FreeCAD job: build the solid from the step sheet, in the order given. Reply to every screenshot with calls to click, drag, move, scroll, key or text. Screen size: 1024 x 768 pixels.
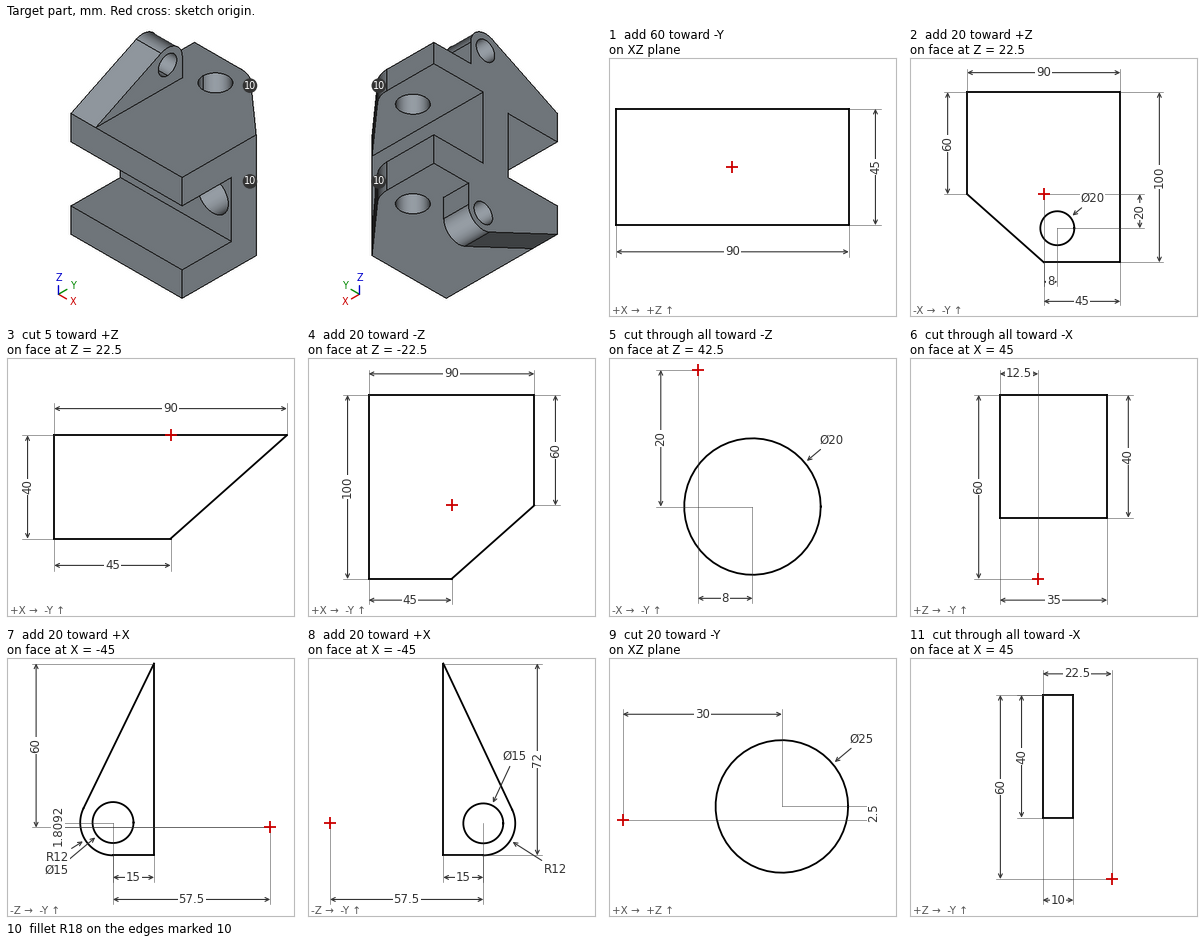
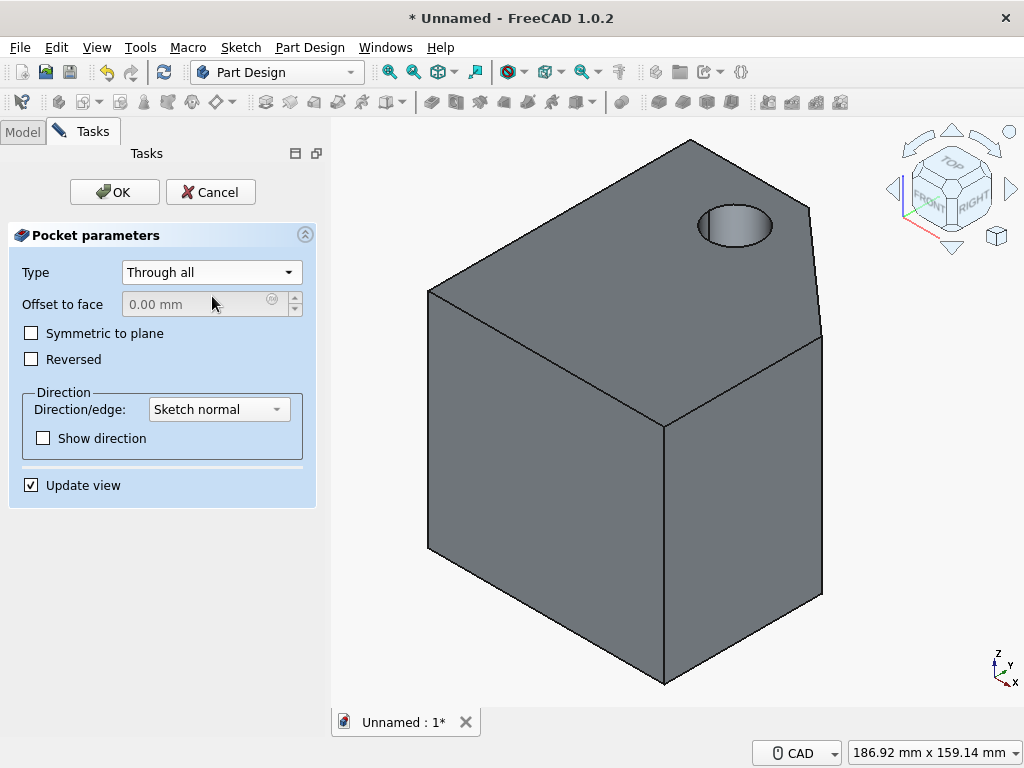
click(115, 192)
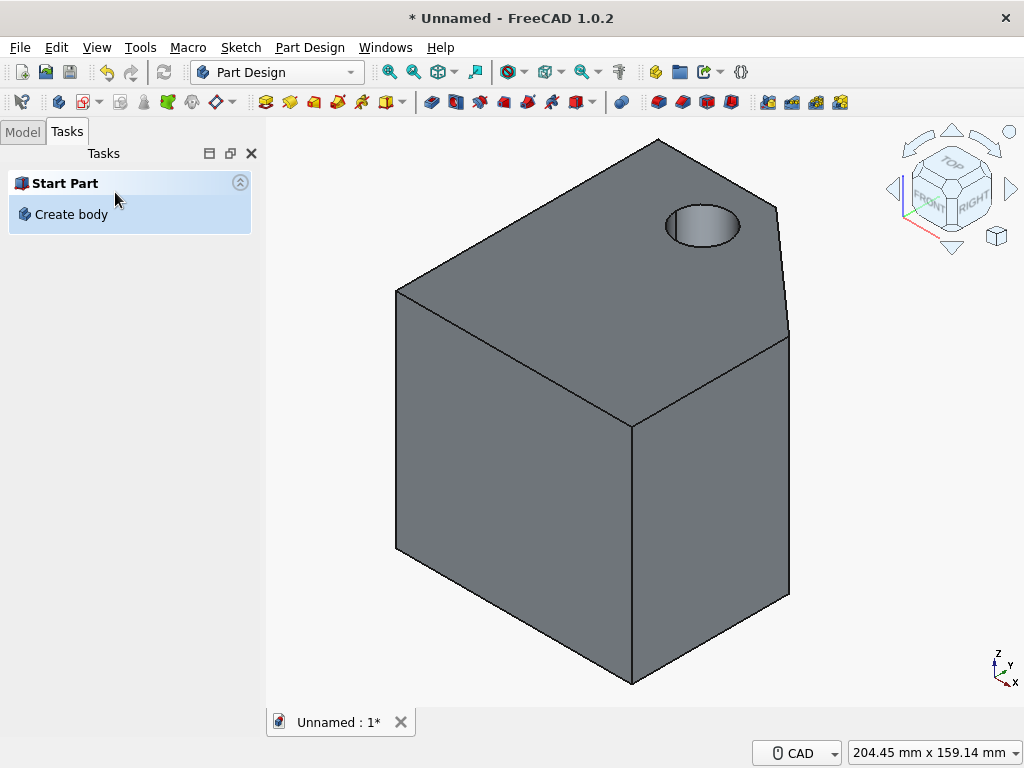
click(711, 546)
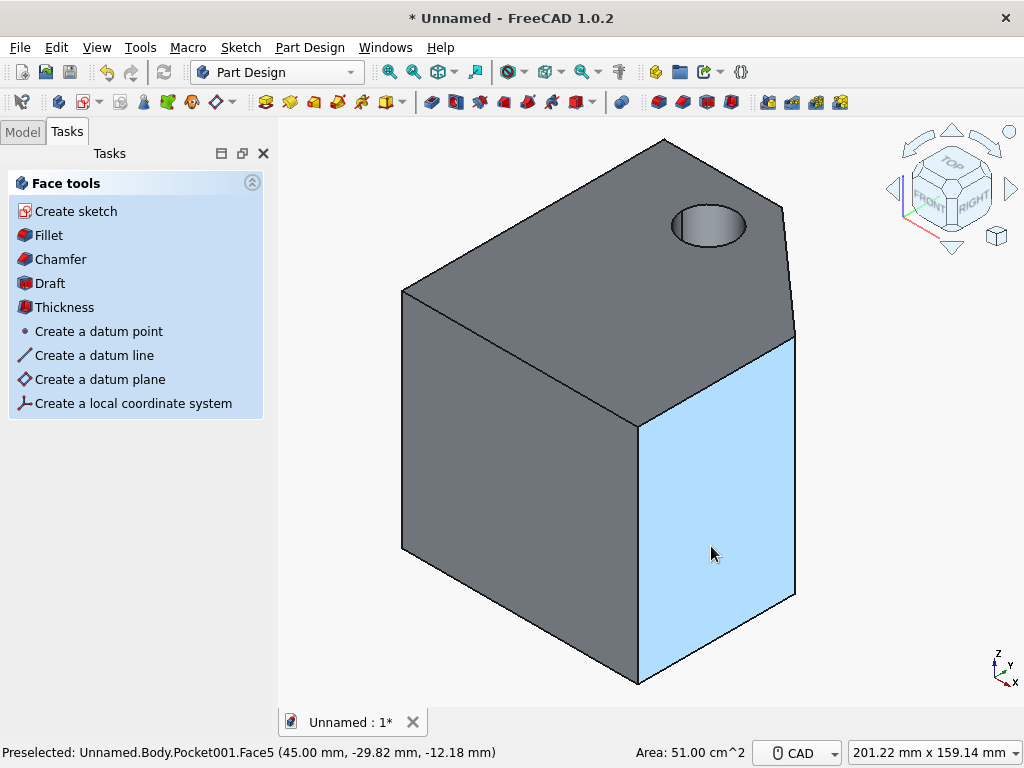
click(84, 102)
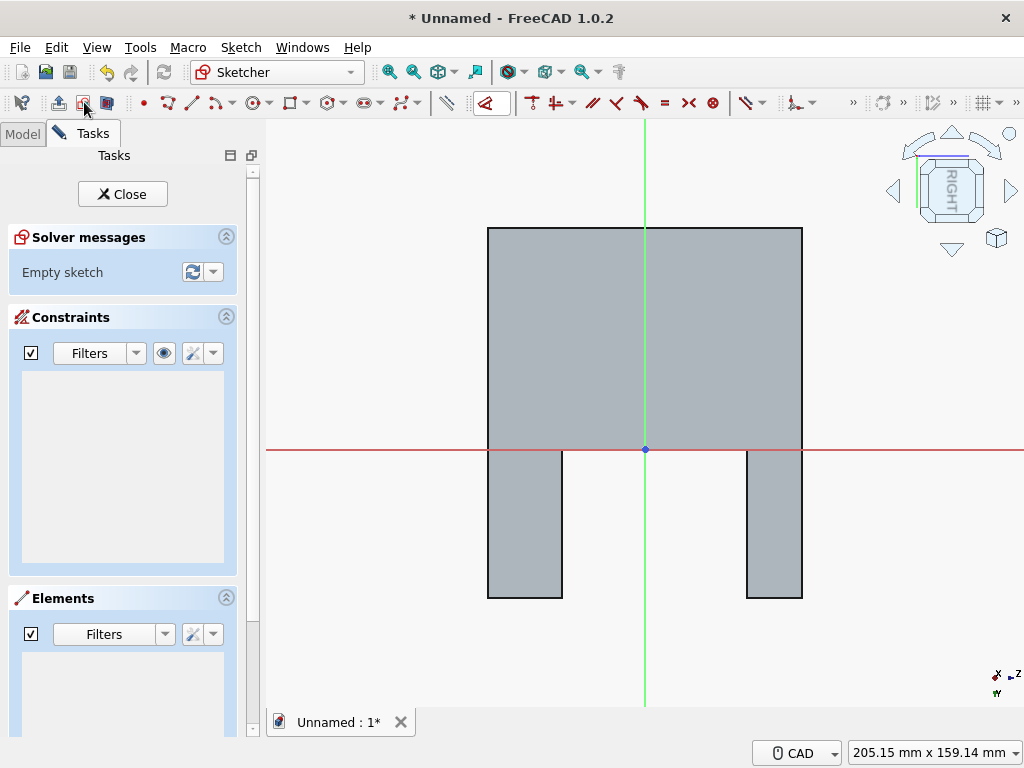
scroll(769, 249, up, 3)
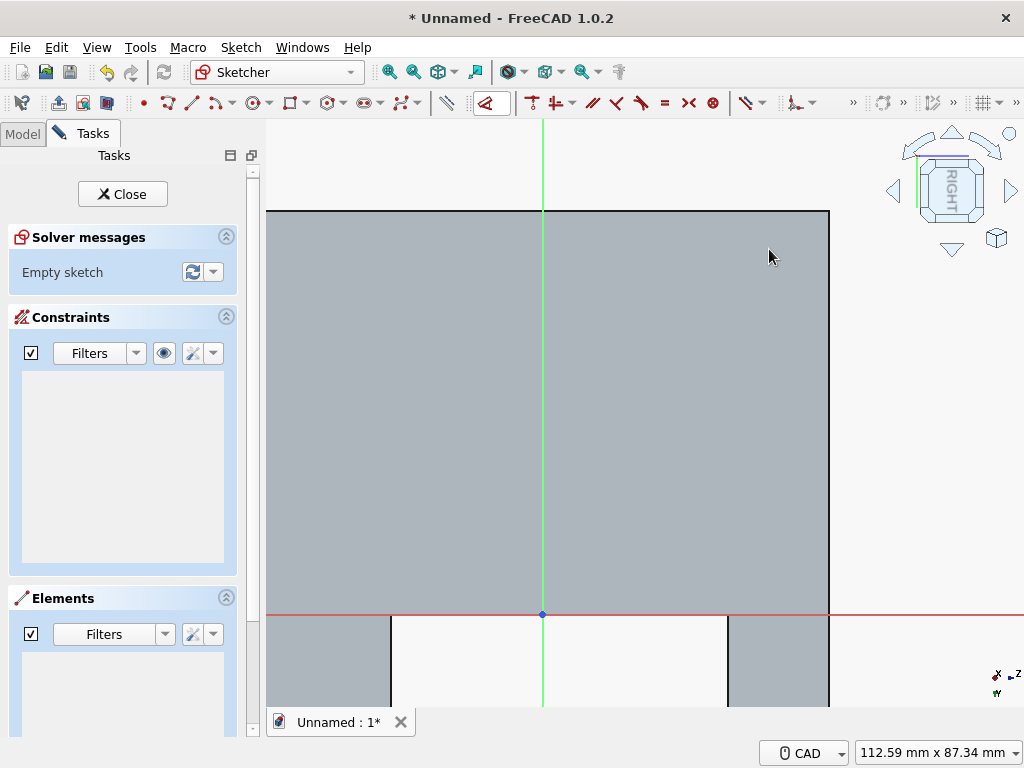
key(g)
key(r)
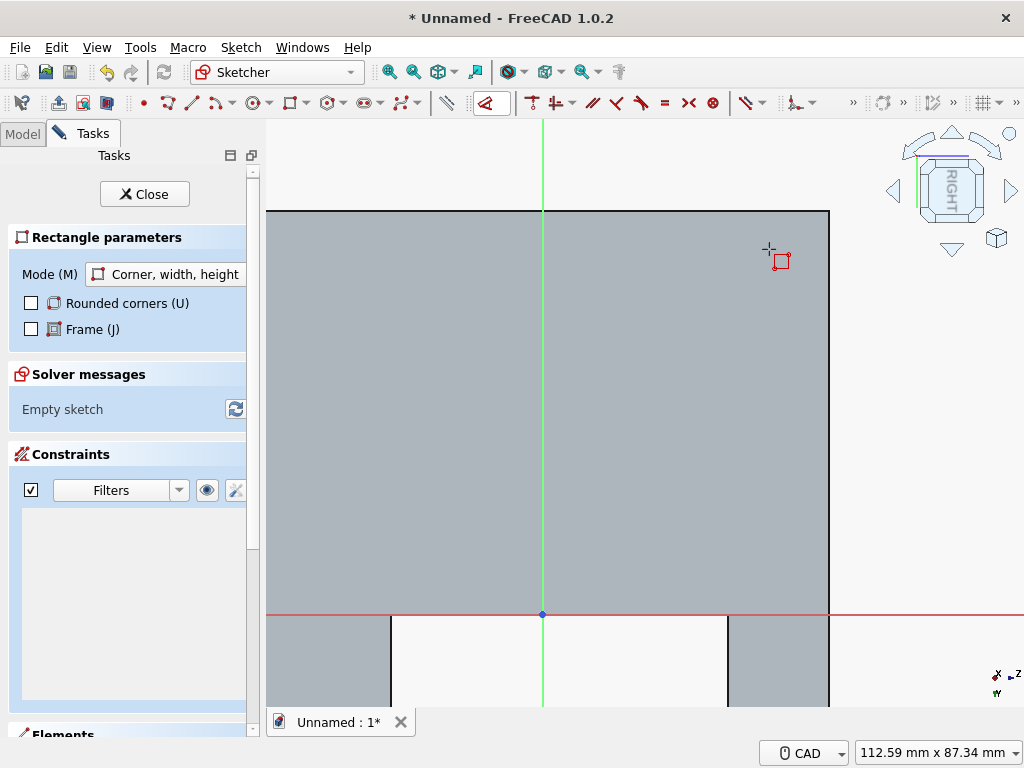
click(458, 211)
move(694, 480)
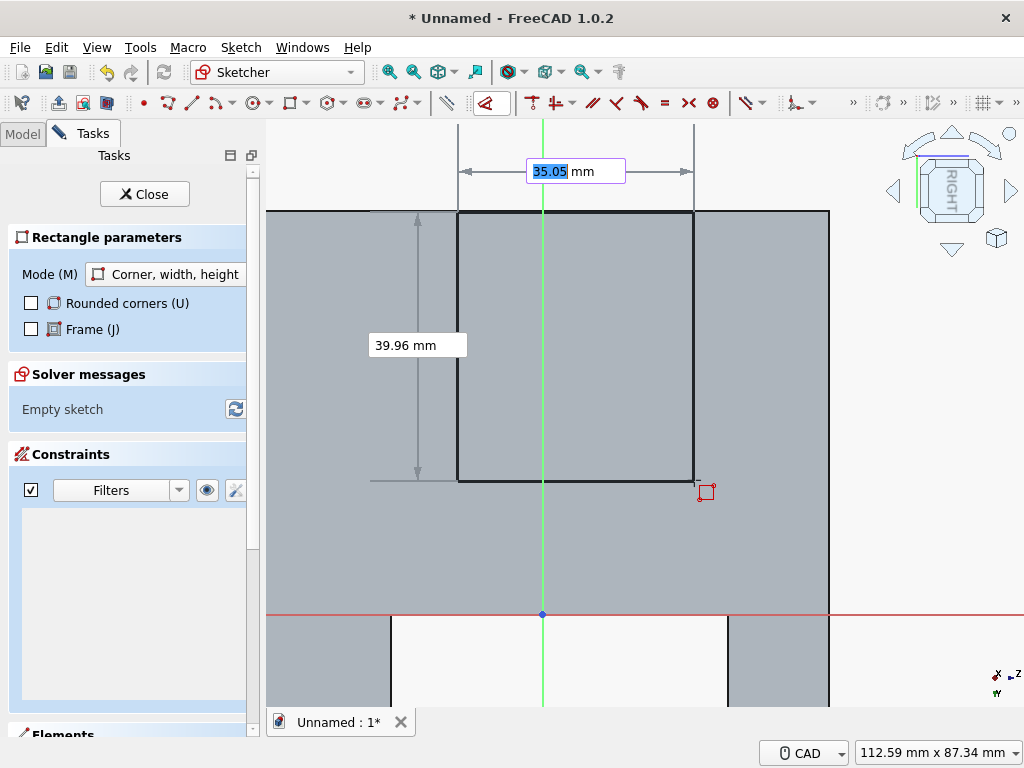
text(35)
key(Tab)
text(40)
key(Return)
key(Escape)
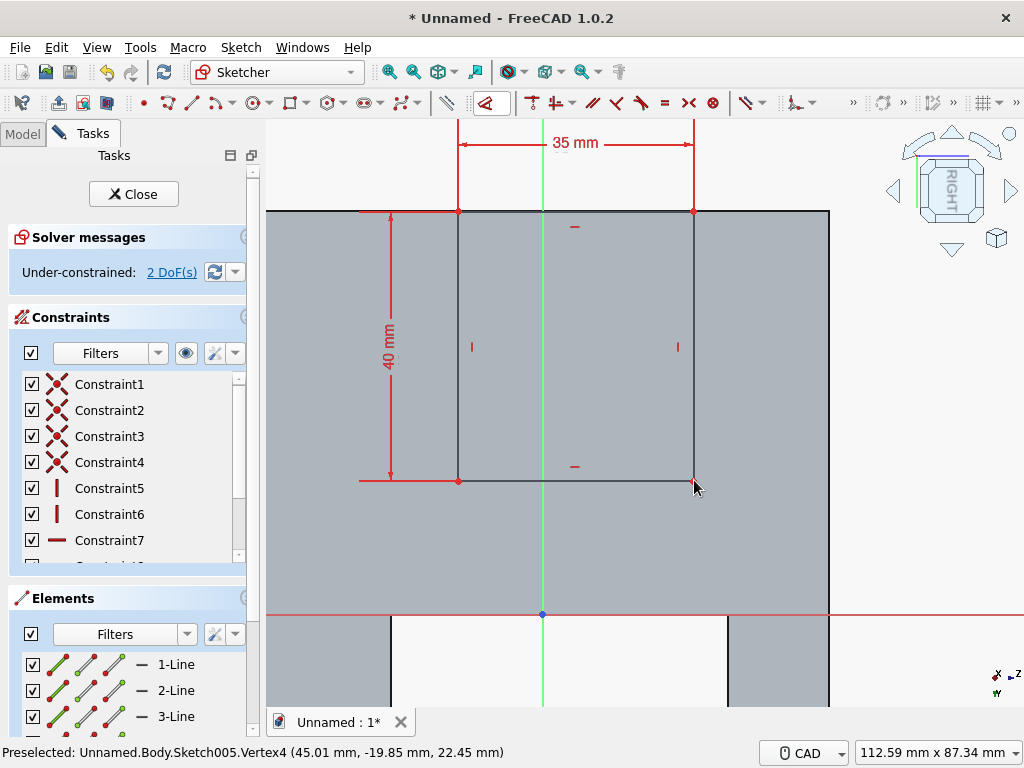
click(458, 212)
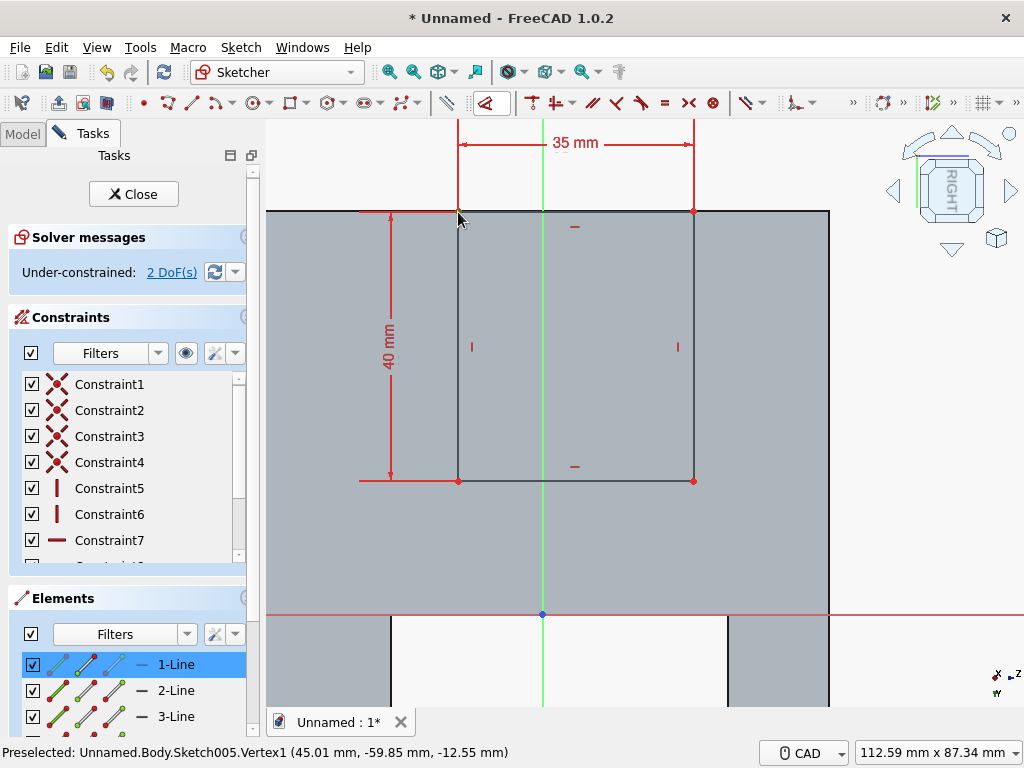
key(i)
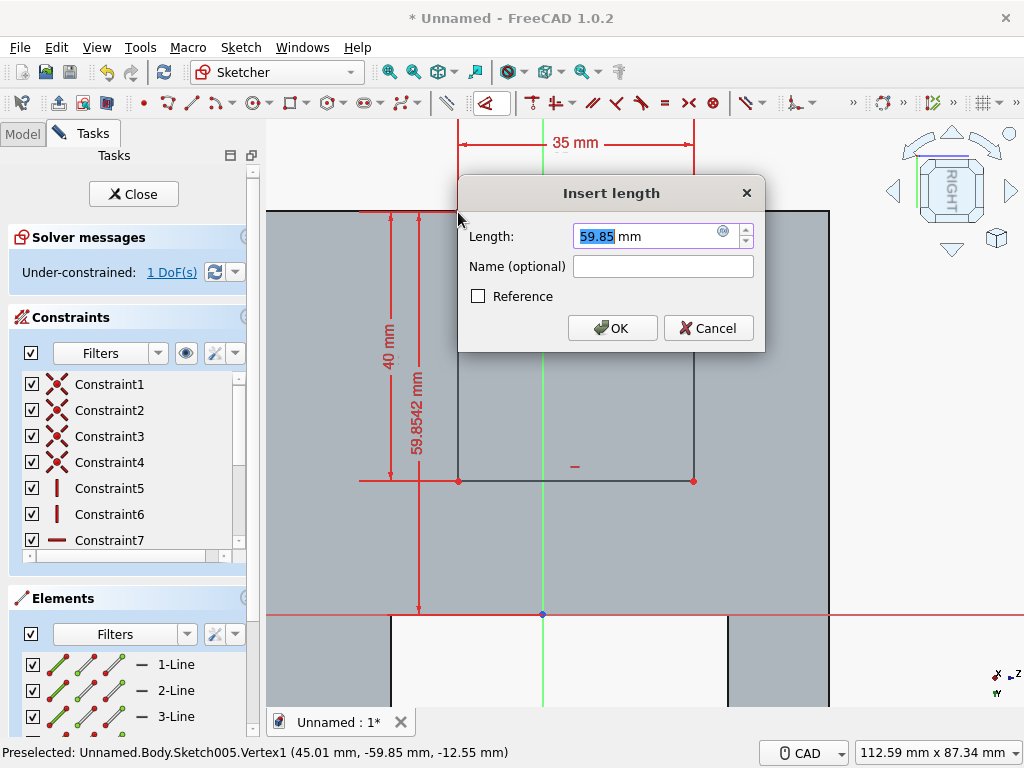
text(60)
key(Return)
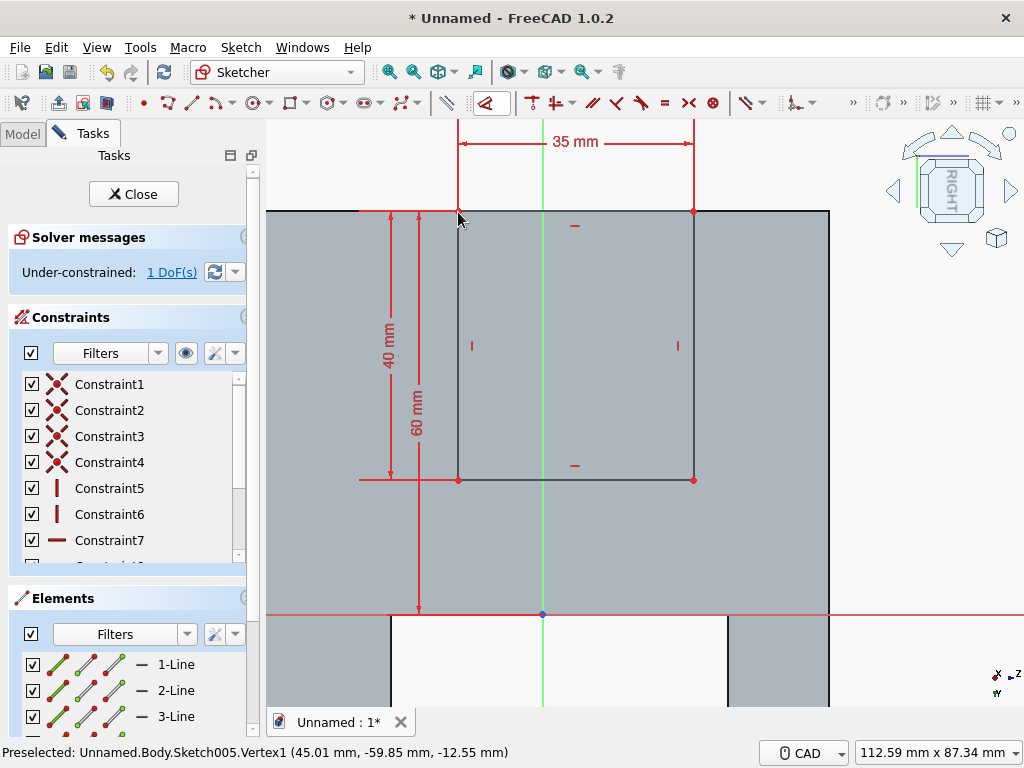
click(458, 211)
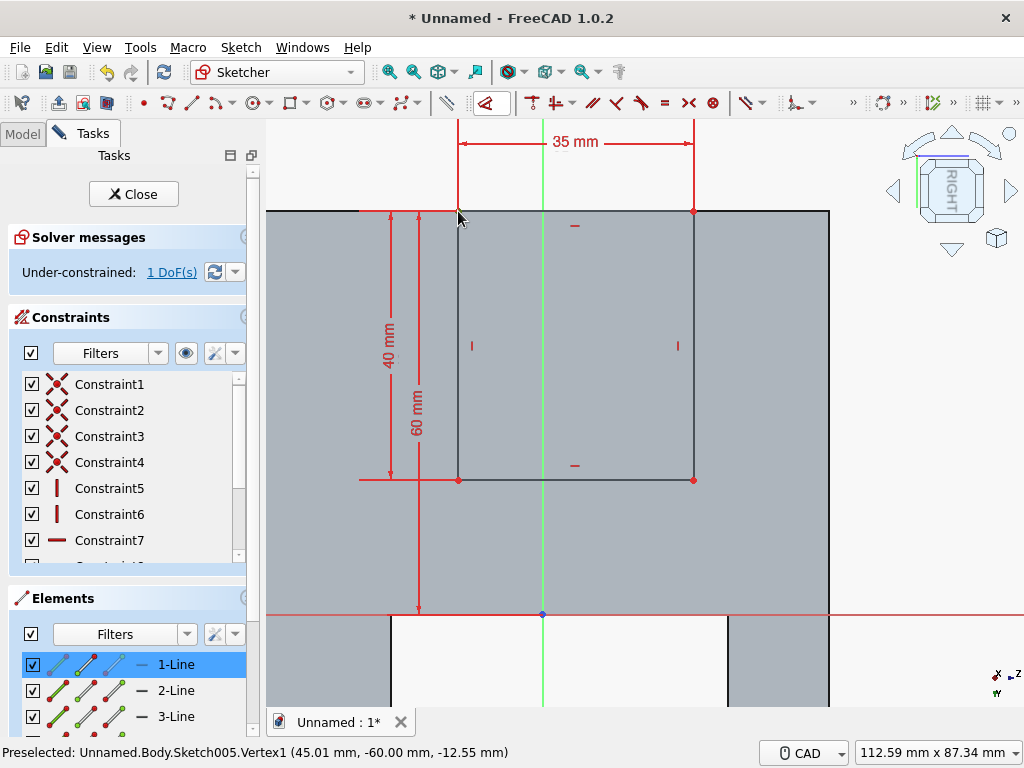
key(l)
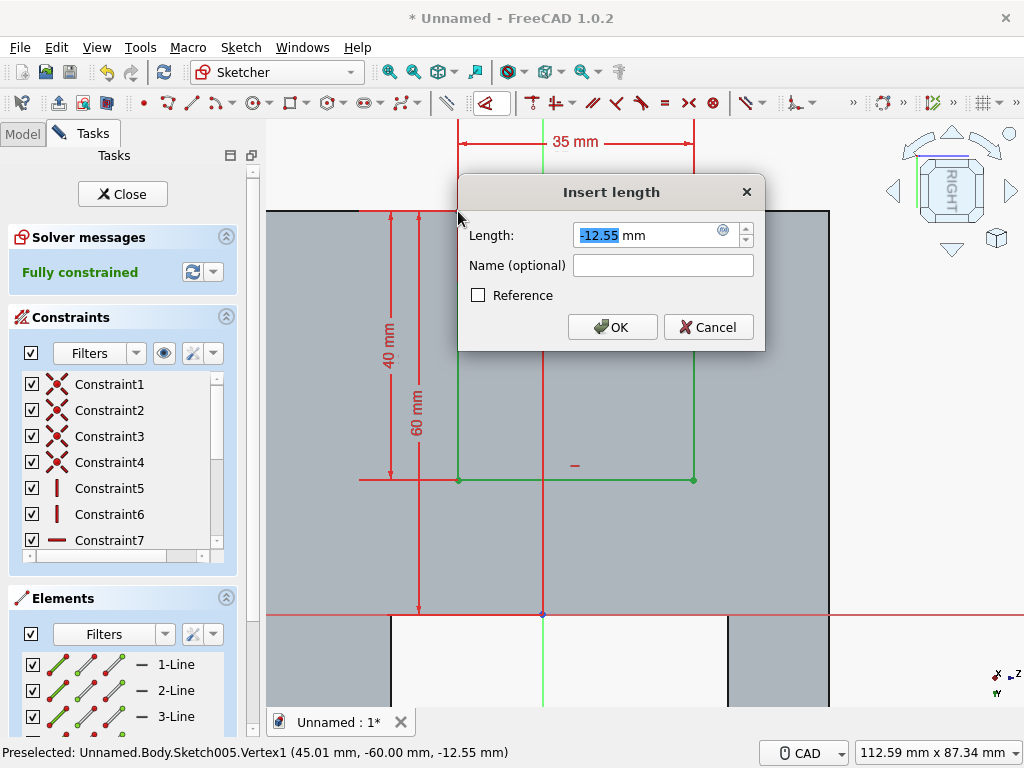
text(-12.5)
key(Return)